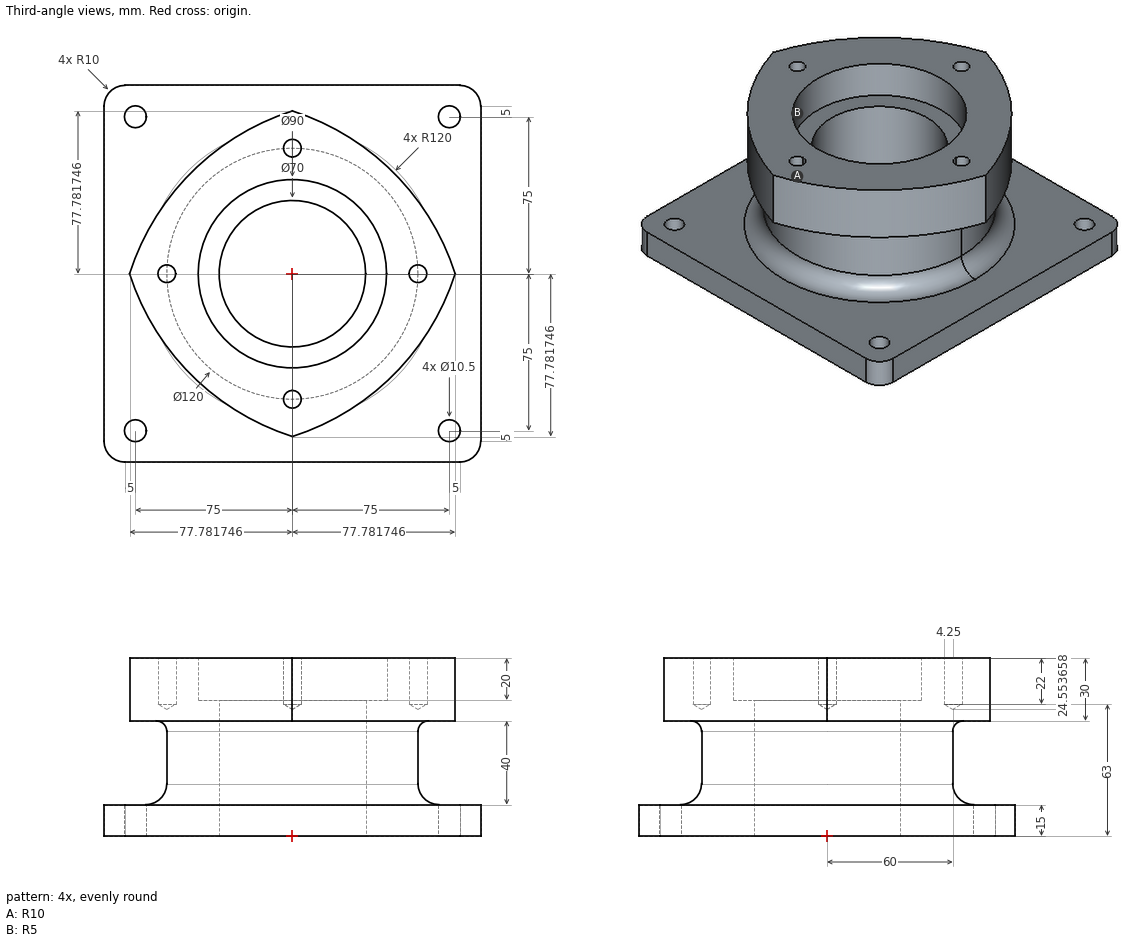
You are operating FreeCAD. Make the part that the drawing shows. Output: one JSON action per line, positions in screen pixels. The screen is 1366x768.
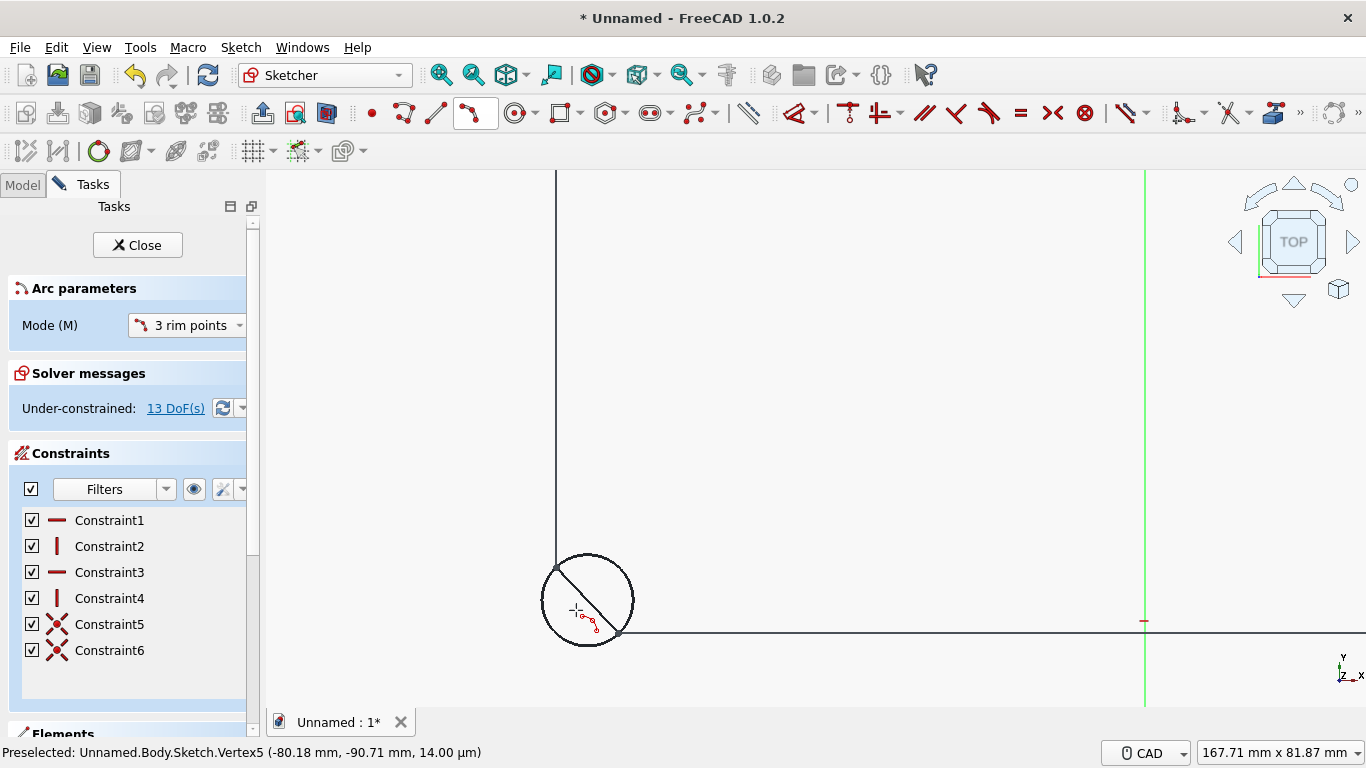
{"action": "left_click", "coordinate": [574, 610]}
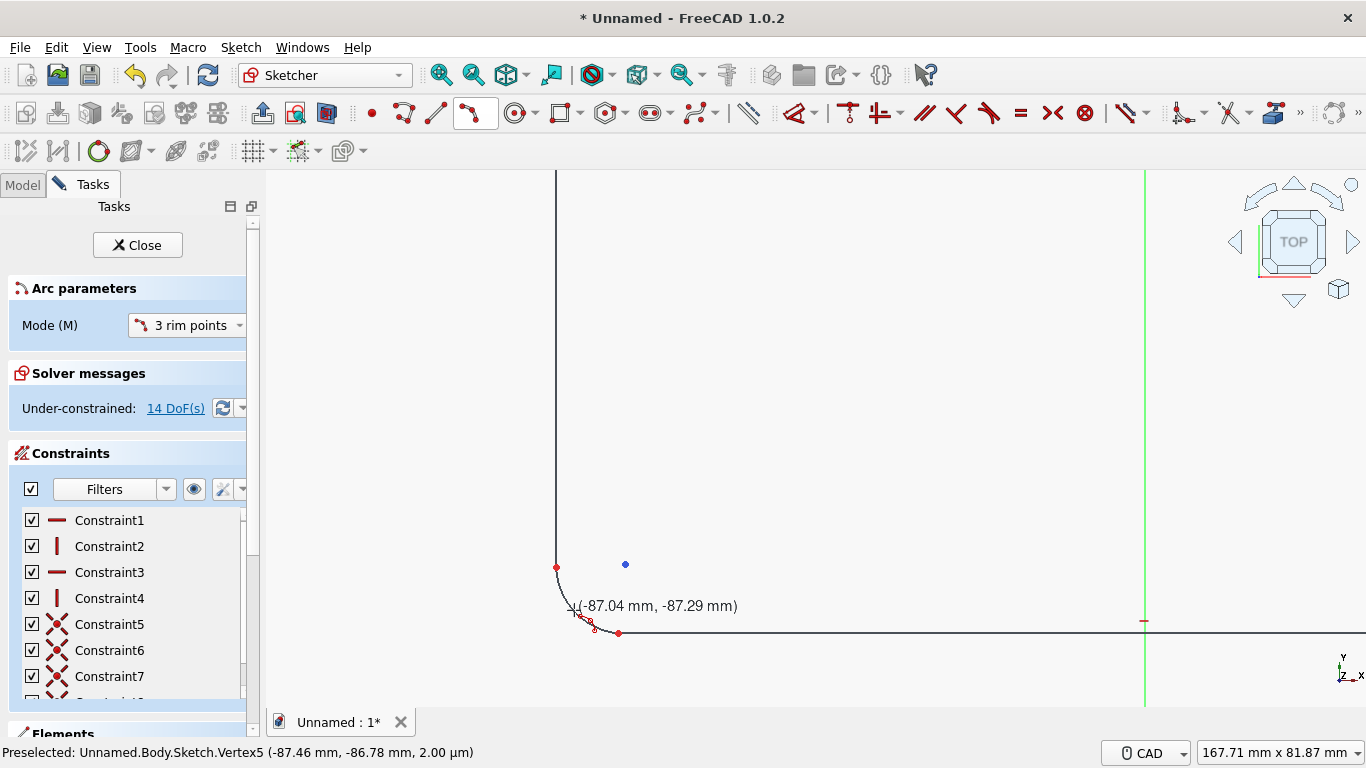
{"action": "scroll", "coordinate": [576, 611], "scroll_direction": "down", "scroll_amount": 6}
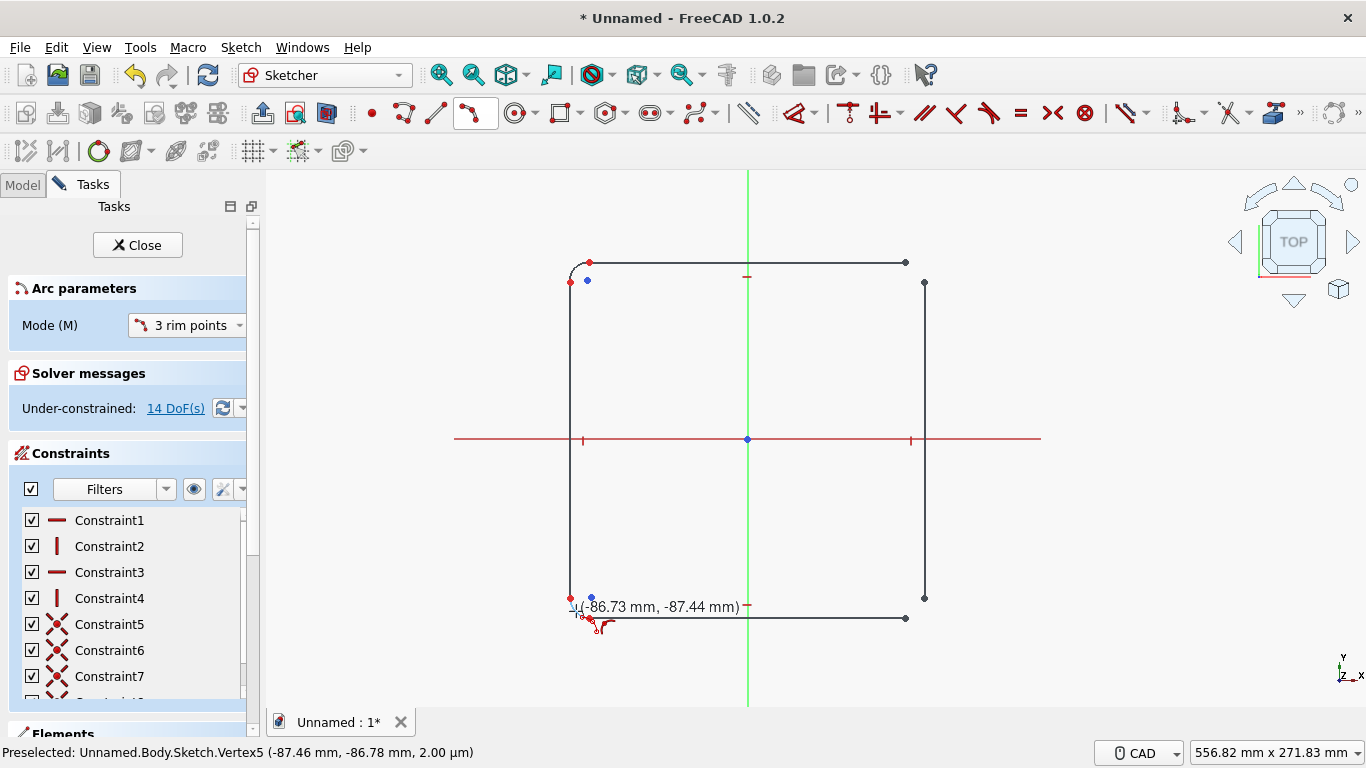
{"action": "left_click", "coordinate": [906, 618]}
{"action": "left_click", "coordinate": [925, 598]}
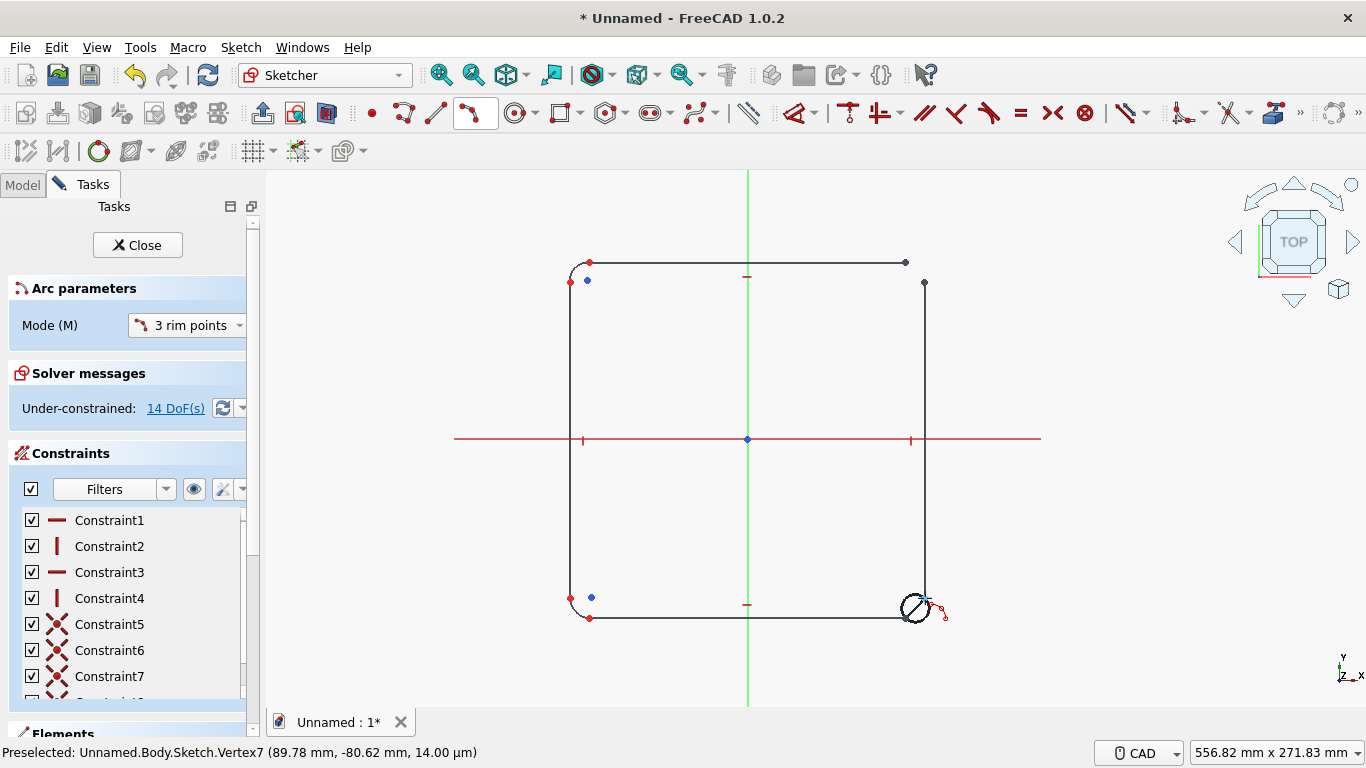
{"action": "scroll", "coordinate": [920, 611], "scroll_direction": "up", "scroll_amount": 6}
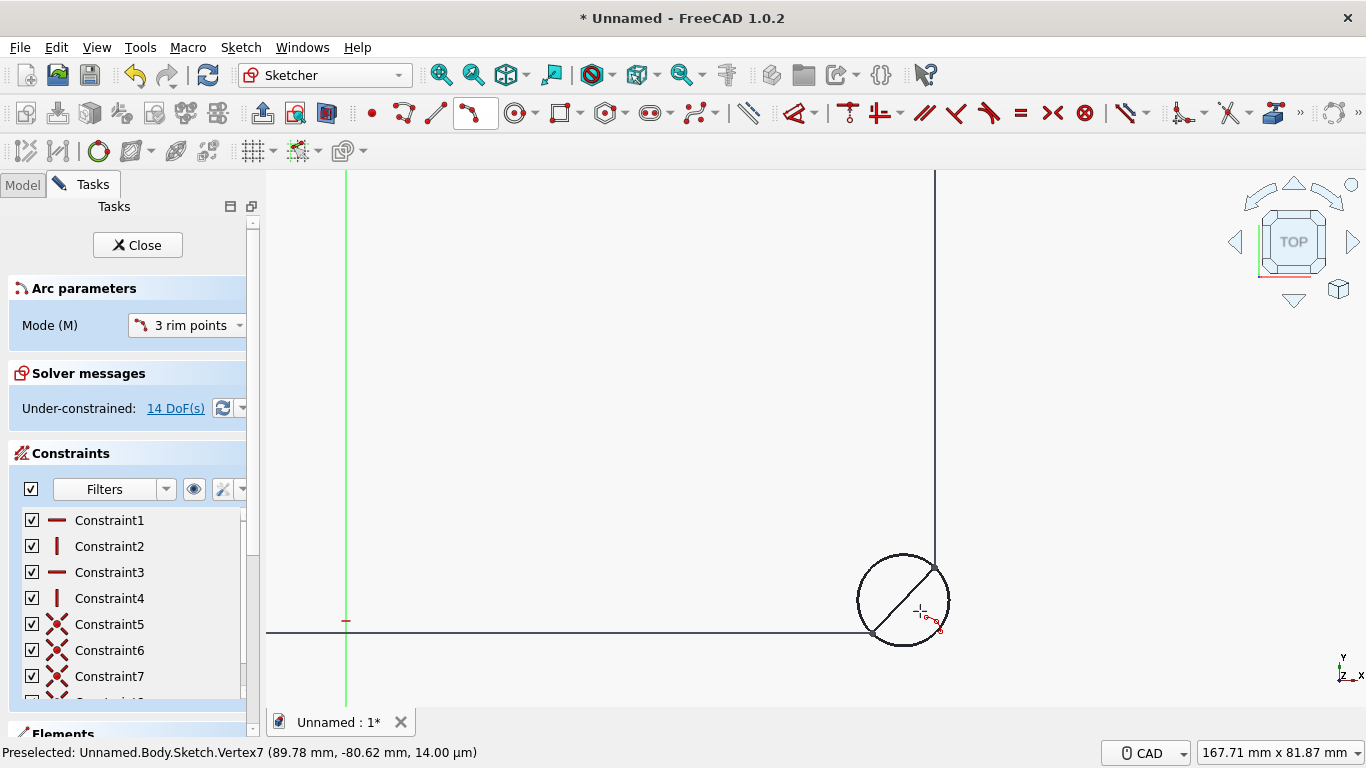
{"action": "left_click", "coordinate": [917, 610]}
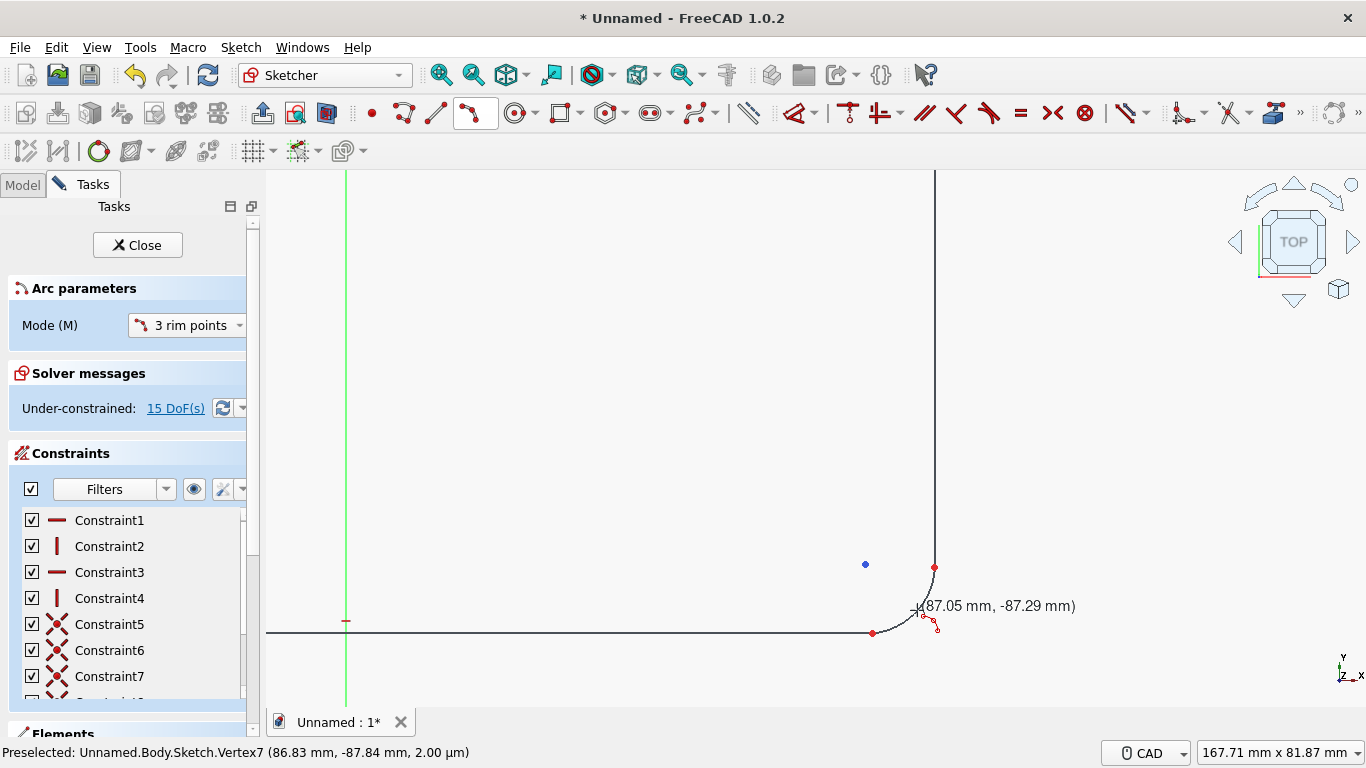
{"action": "scroll", "coordinate": [921, 611], "scroll_direction": "down", "scroll_amount": 6}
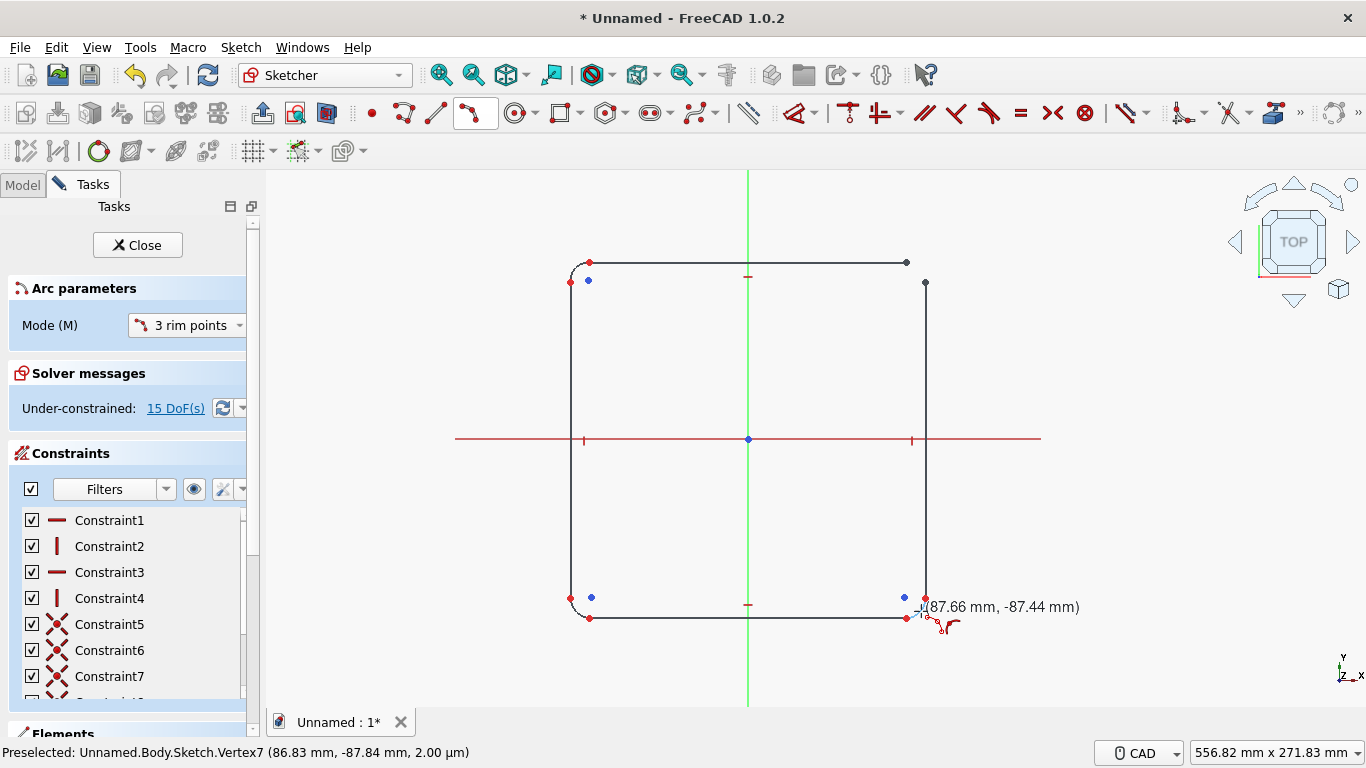
{"action": "left_click", "coordinate": [926, 283]}
{"action": "left_click", "coordinate": [907, 263]}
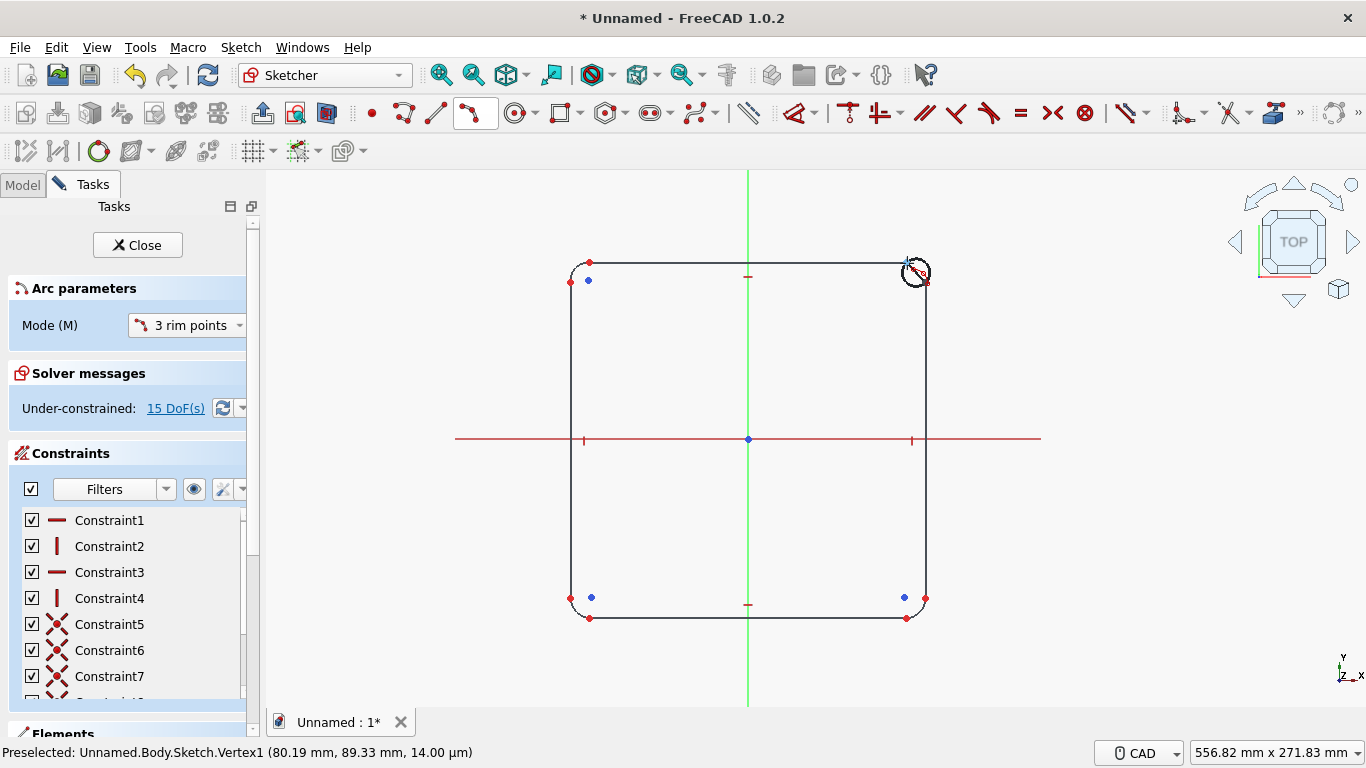
{"action": "scroll", "coordinate": [920, 267], "scroll_direction": "up", "scroll_amount": 6}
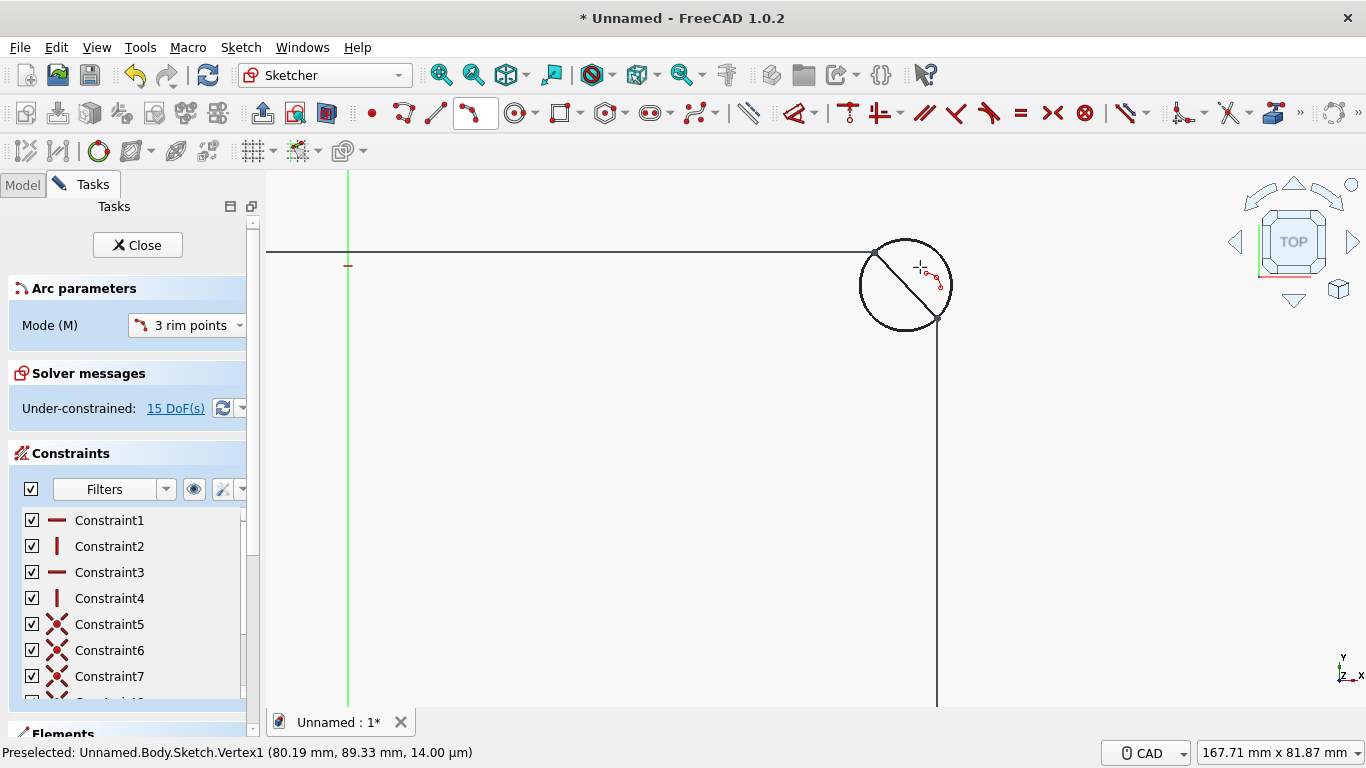
{"action": "left_click", "coordinate": [919, 267]}